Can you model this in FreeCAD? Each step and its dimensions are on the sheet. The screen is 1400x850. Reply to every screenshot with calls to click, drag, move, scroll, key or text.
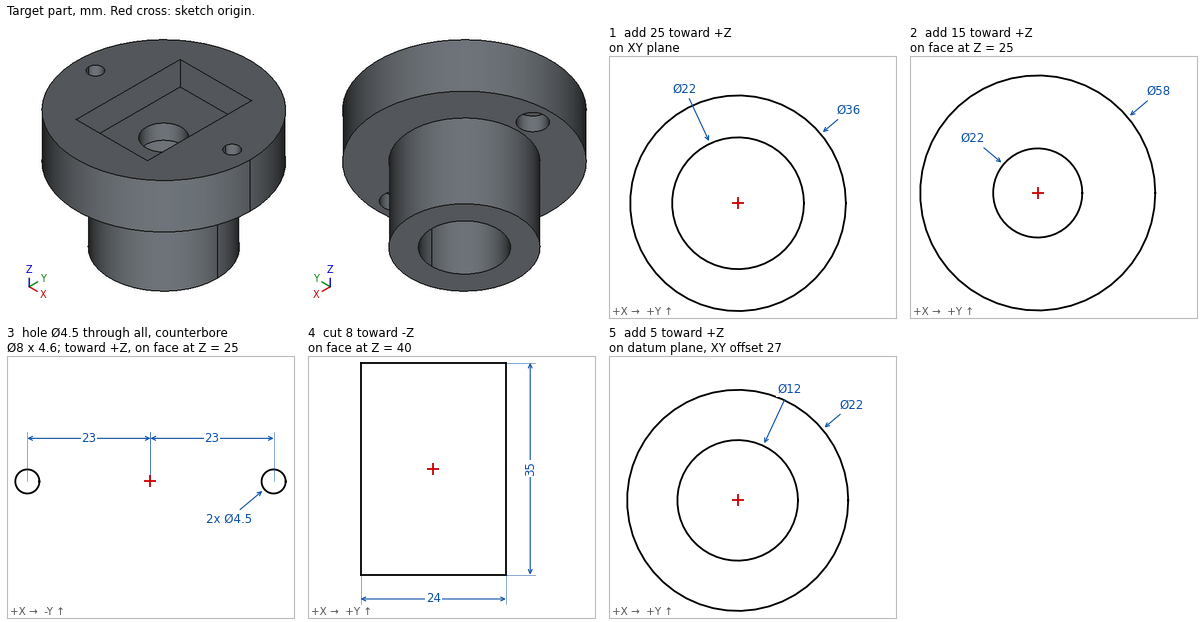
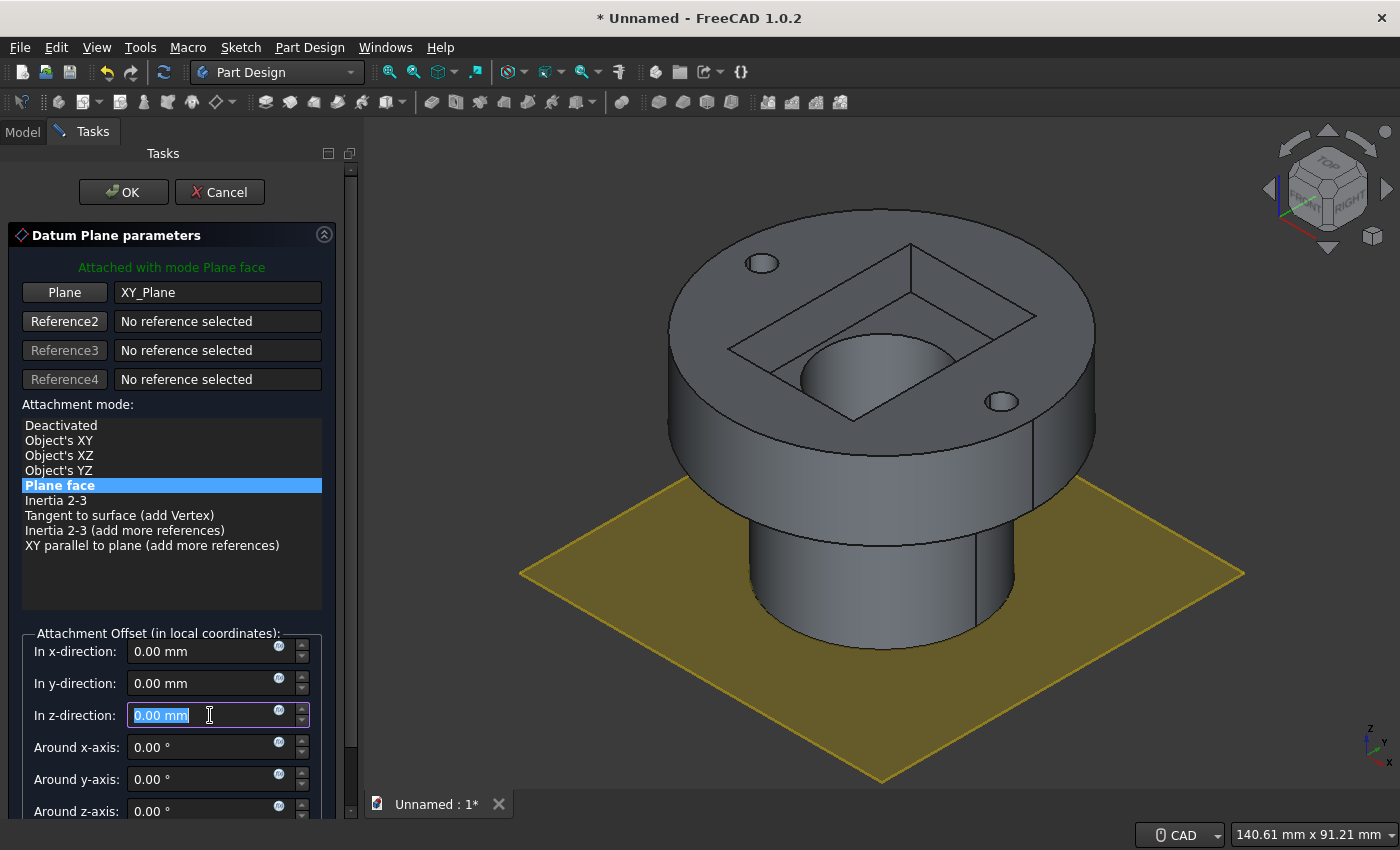
text(27)
key(Tab)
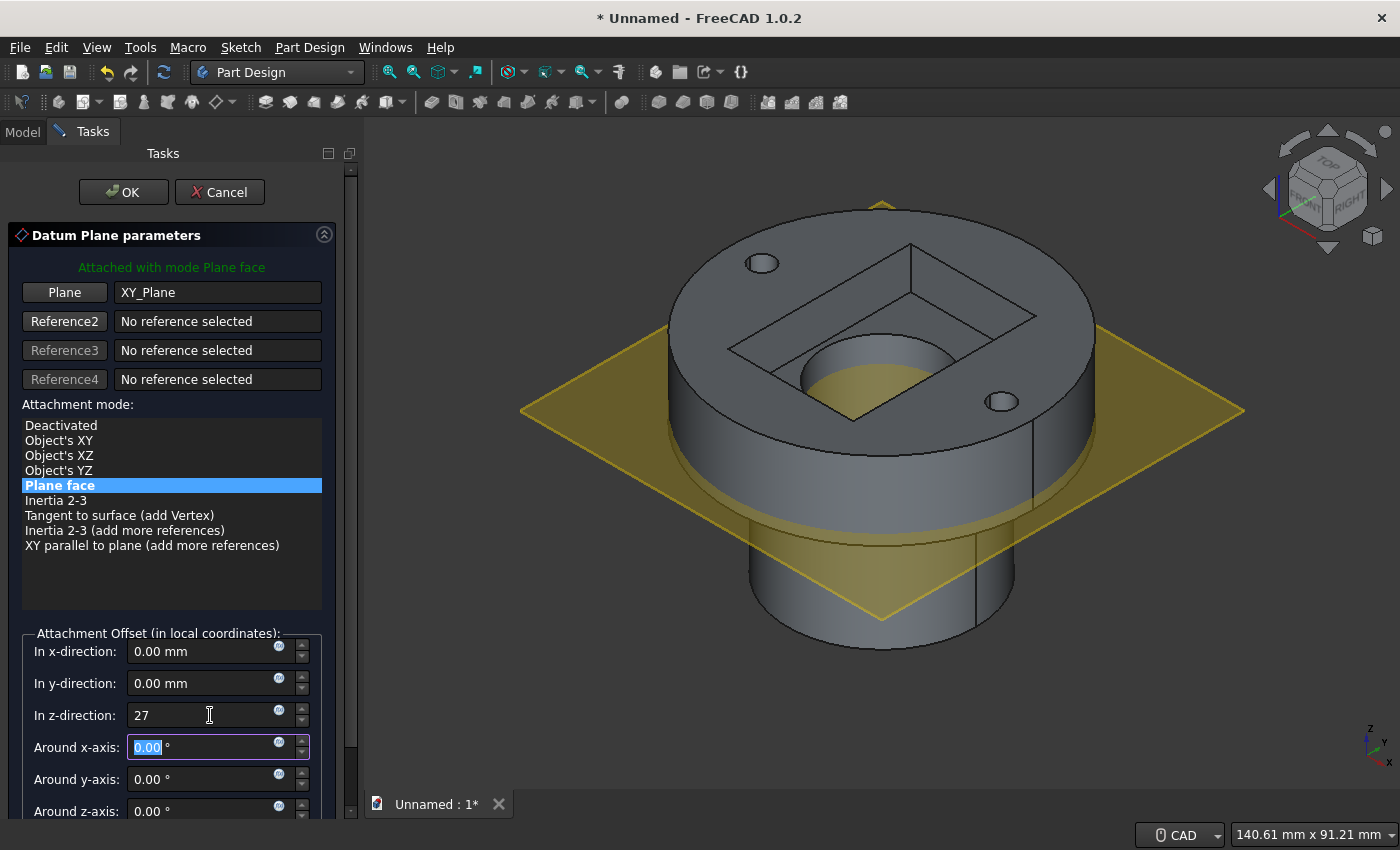
click(124, 192)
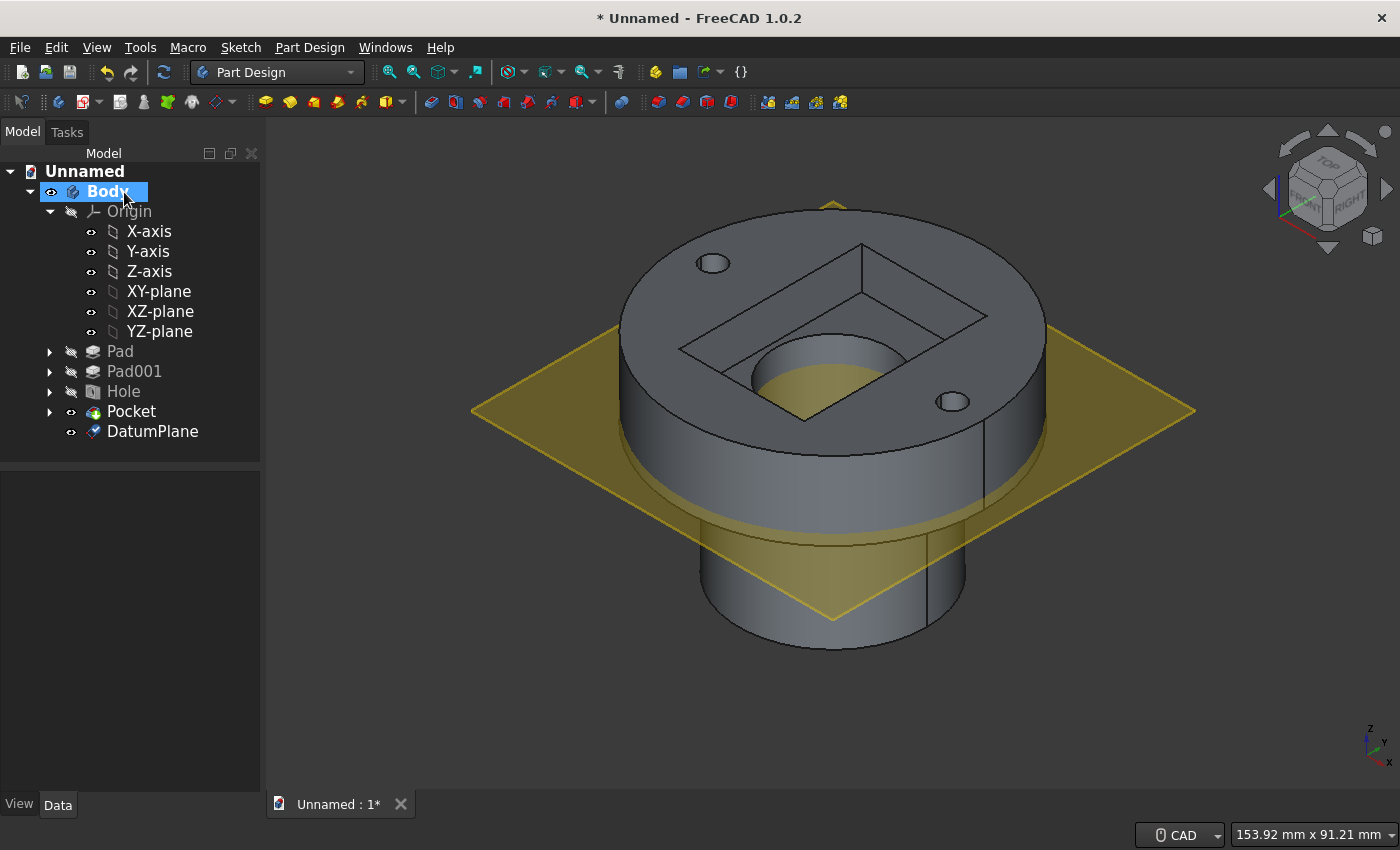
click(116, 432)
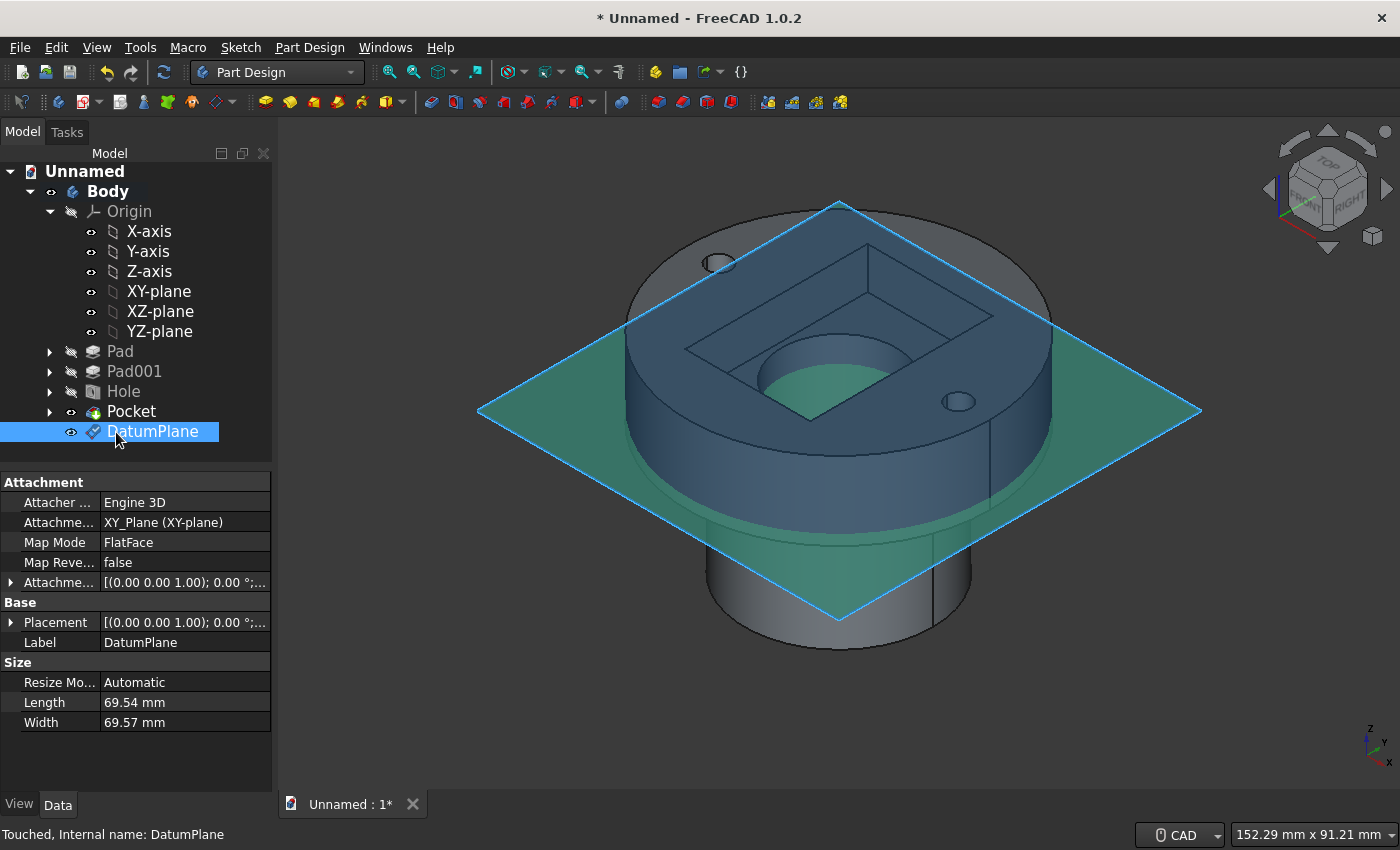
click(84, 102)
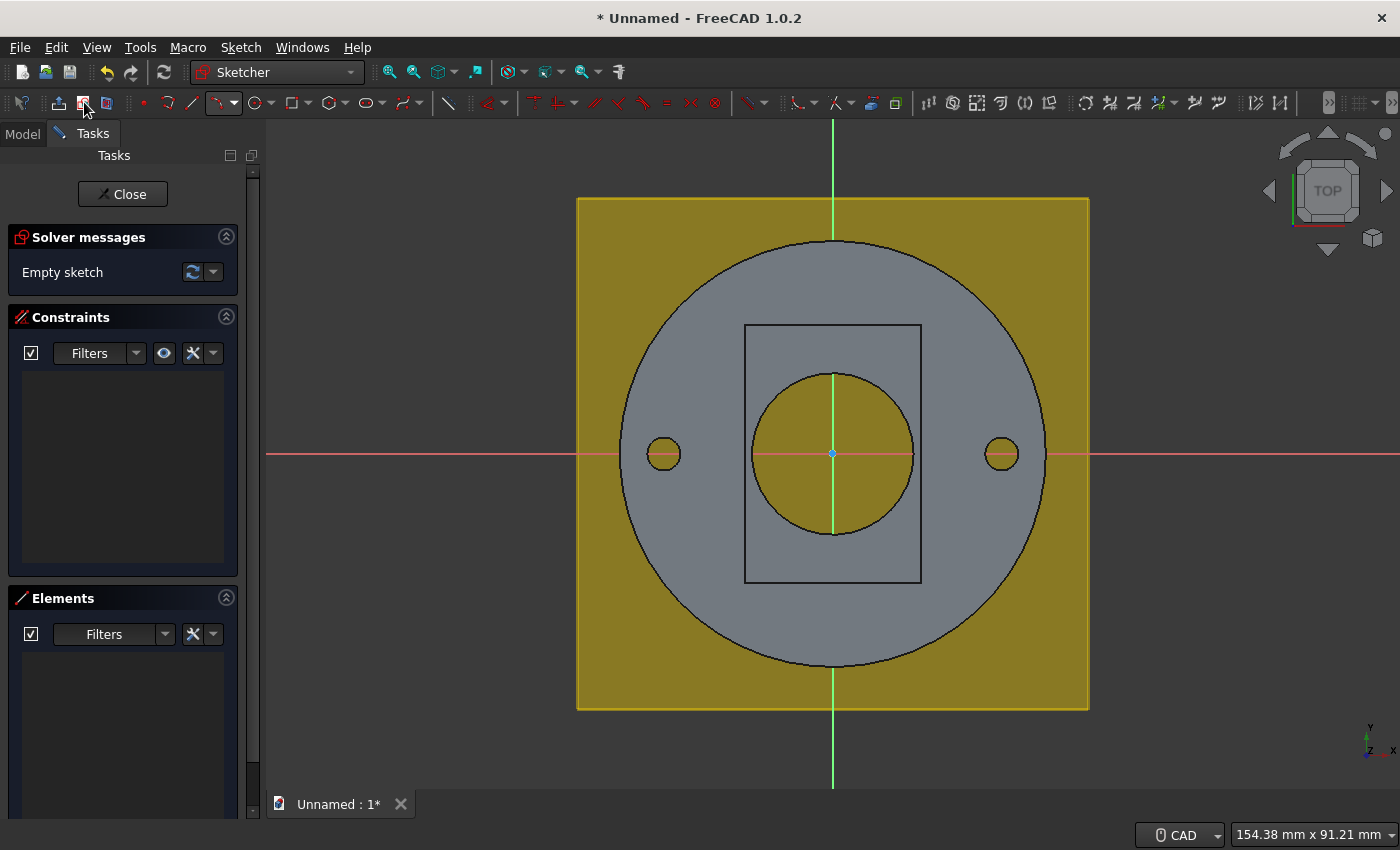
key(q)
key(s)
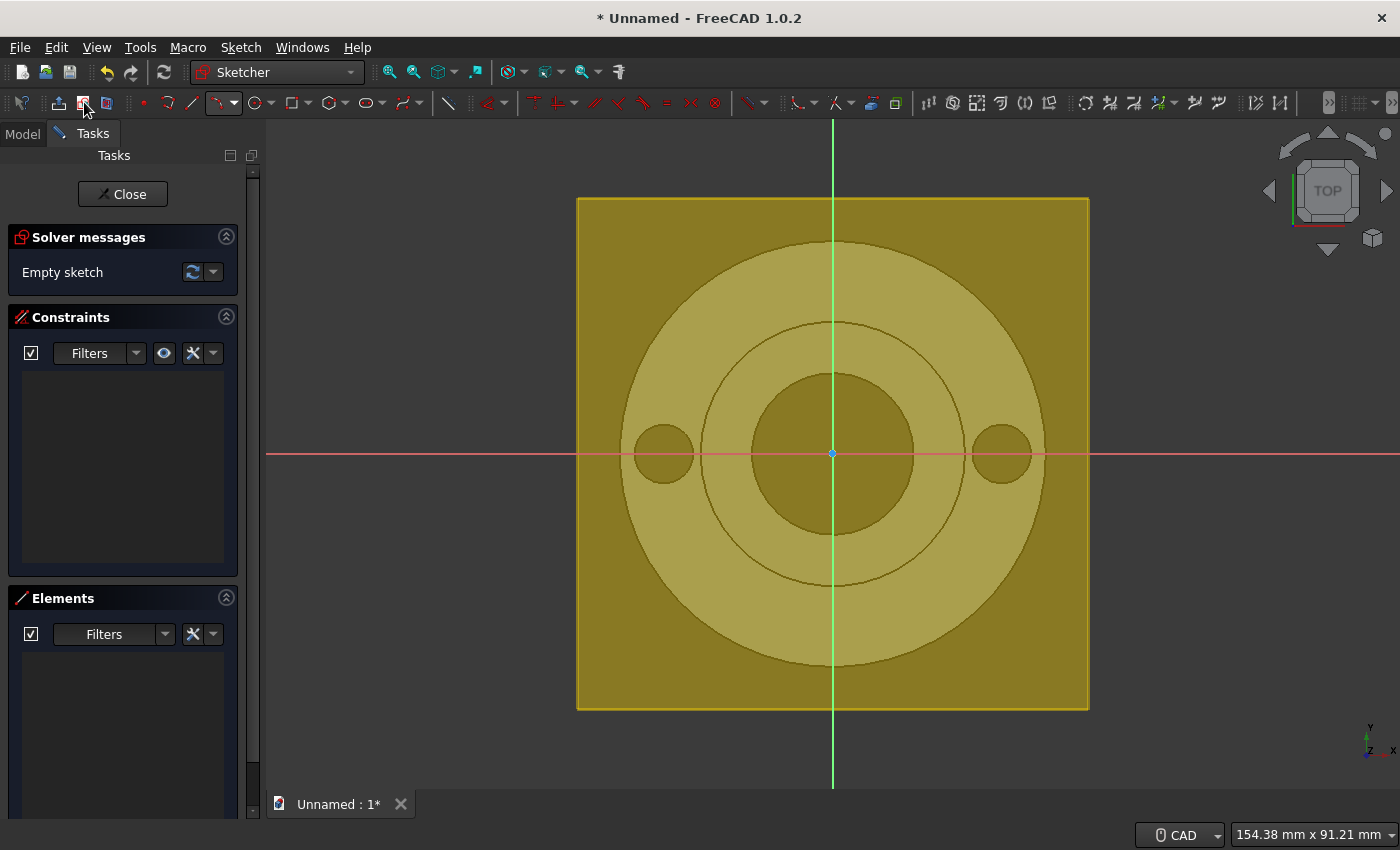
scroll(873, 454, up, 5)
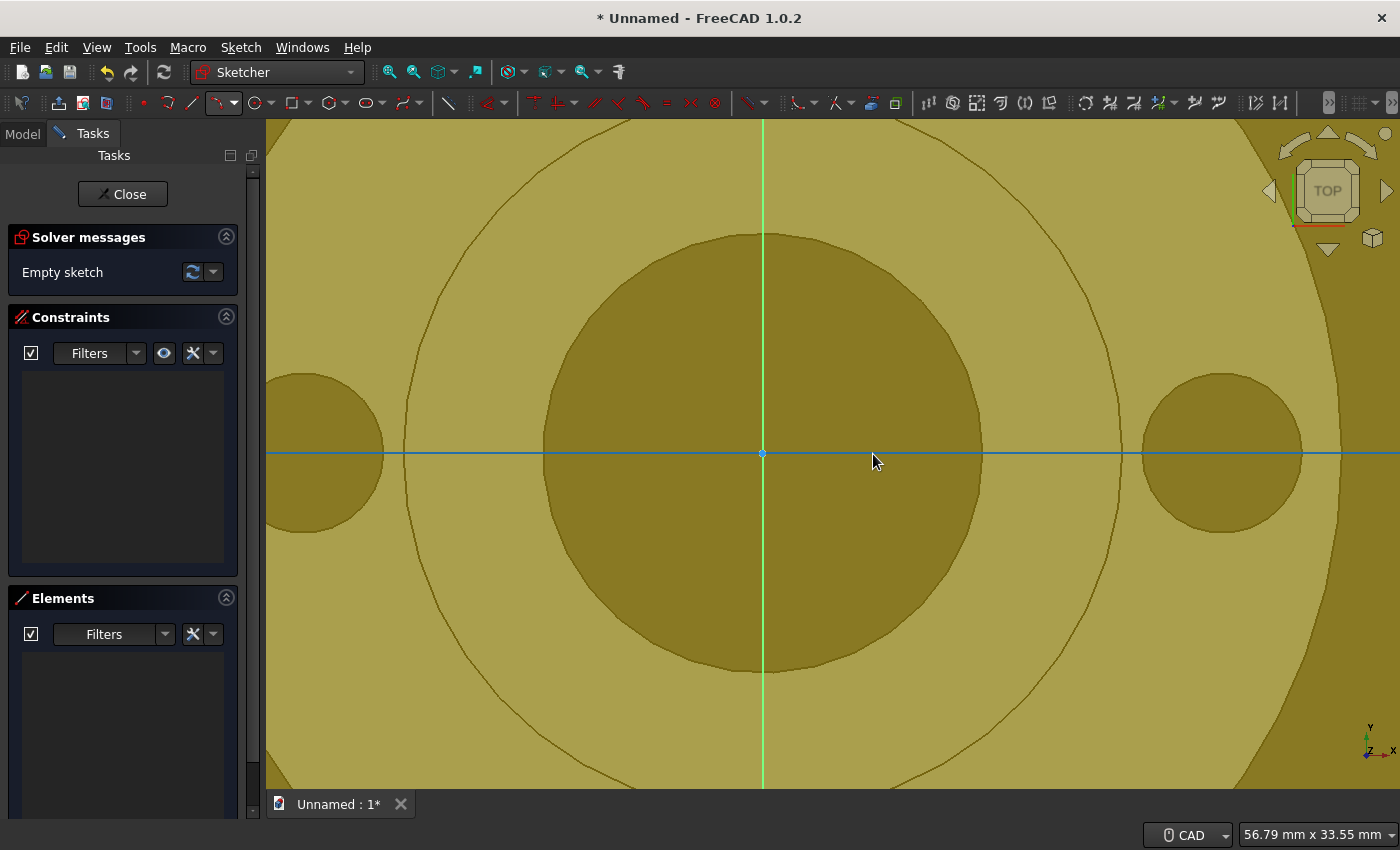
key(g)
key(c)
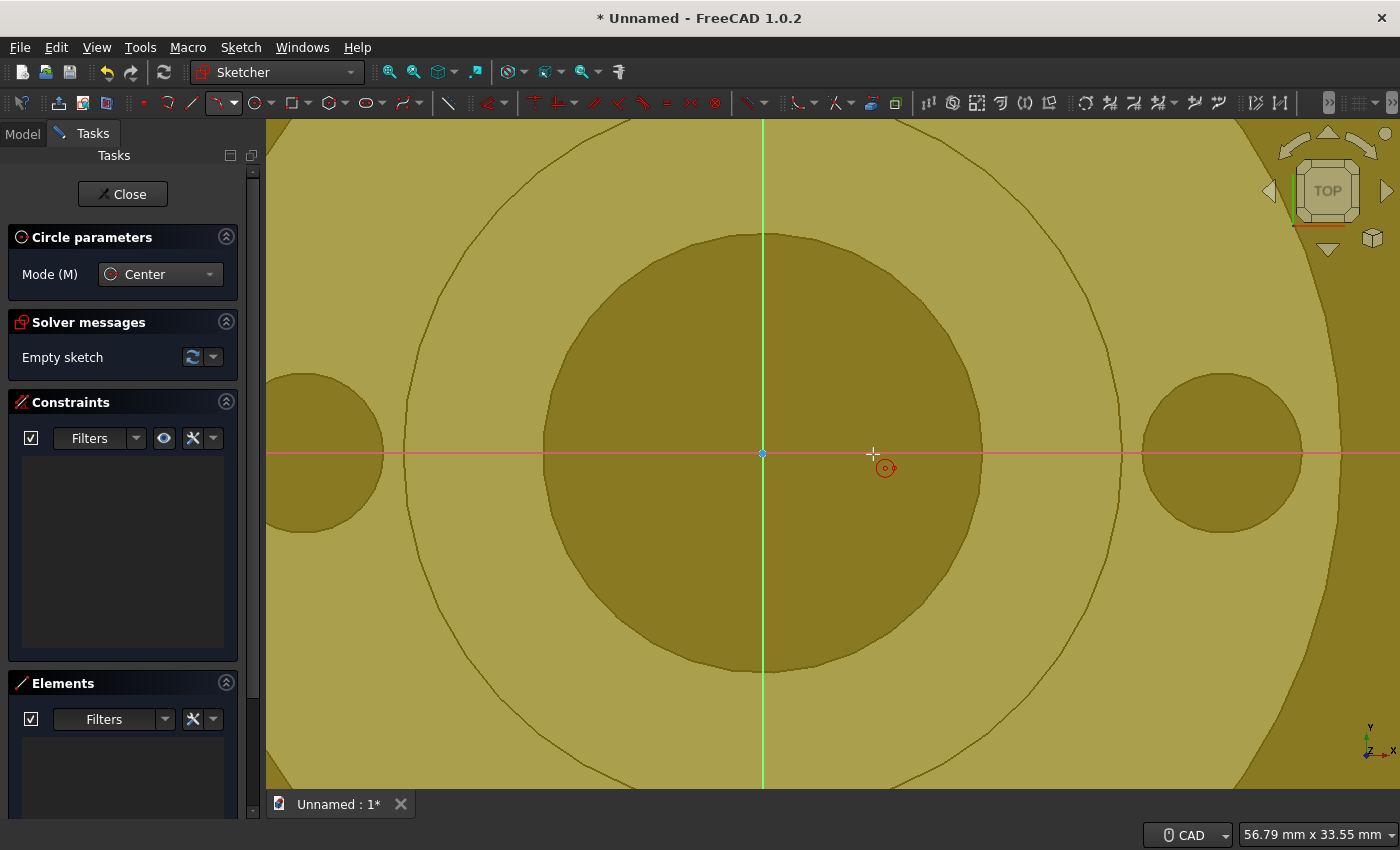
click(763, 453)
click(918, 298)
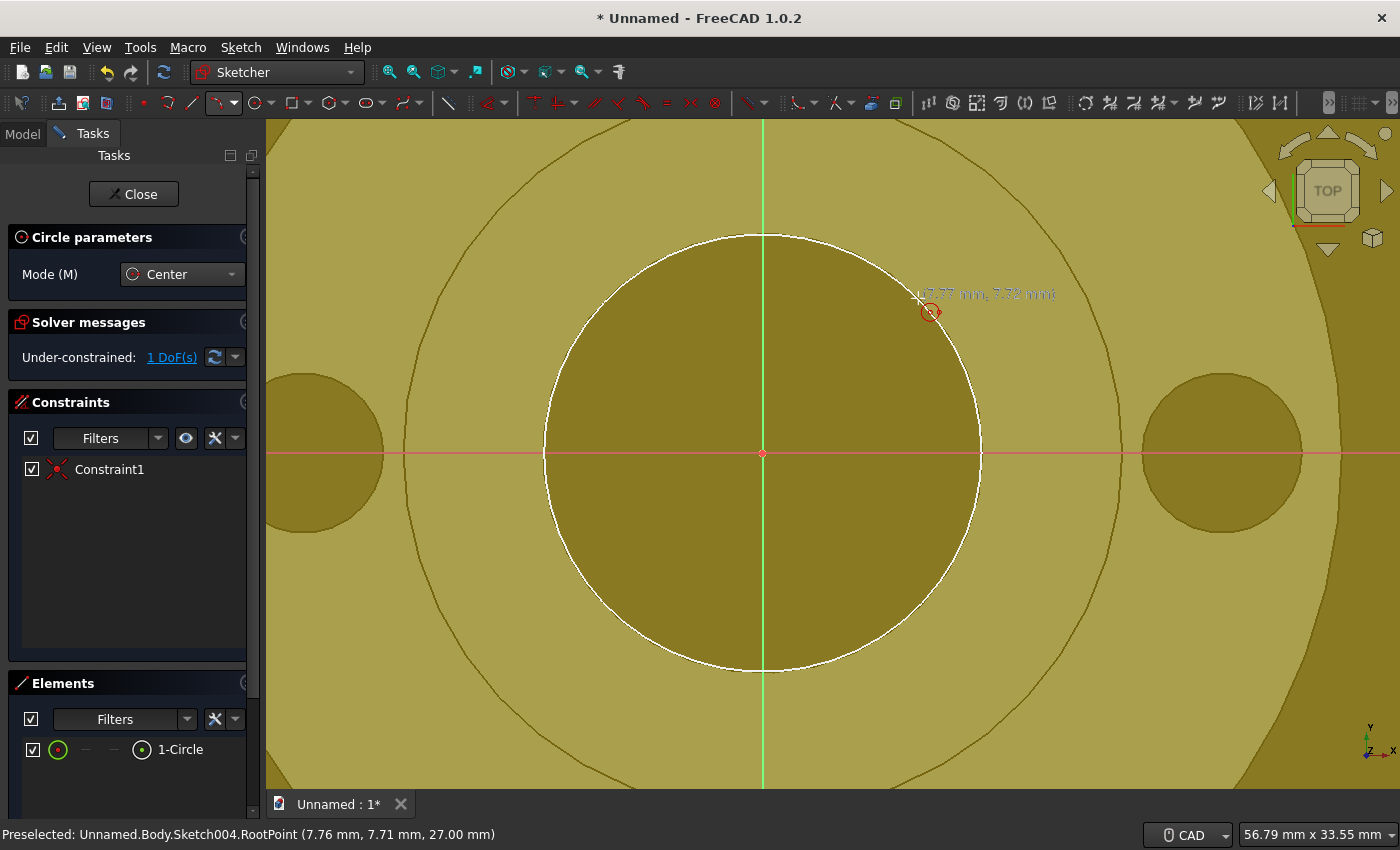
click(763, 453)
click(848, 368)
key(Escape)